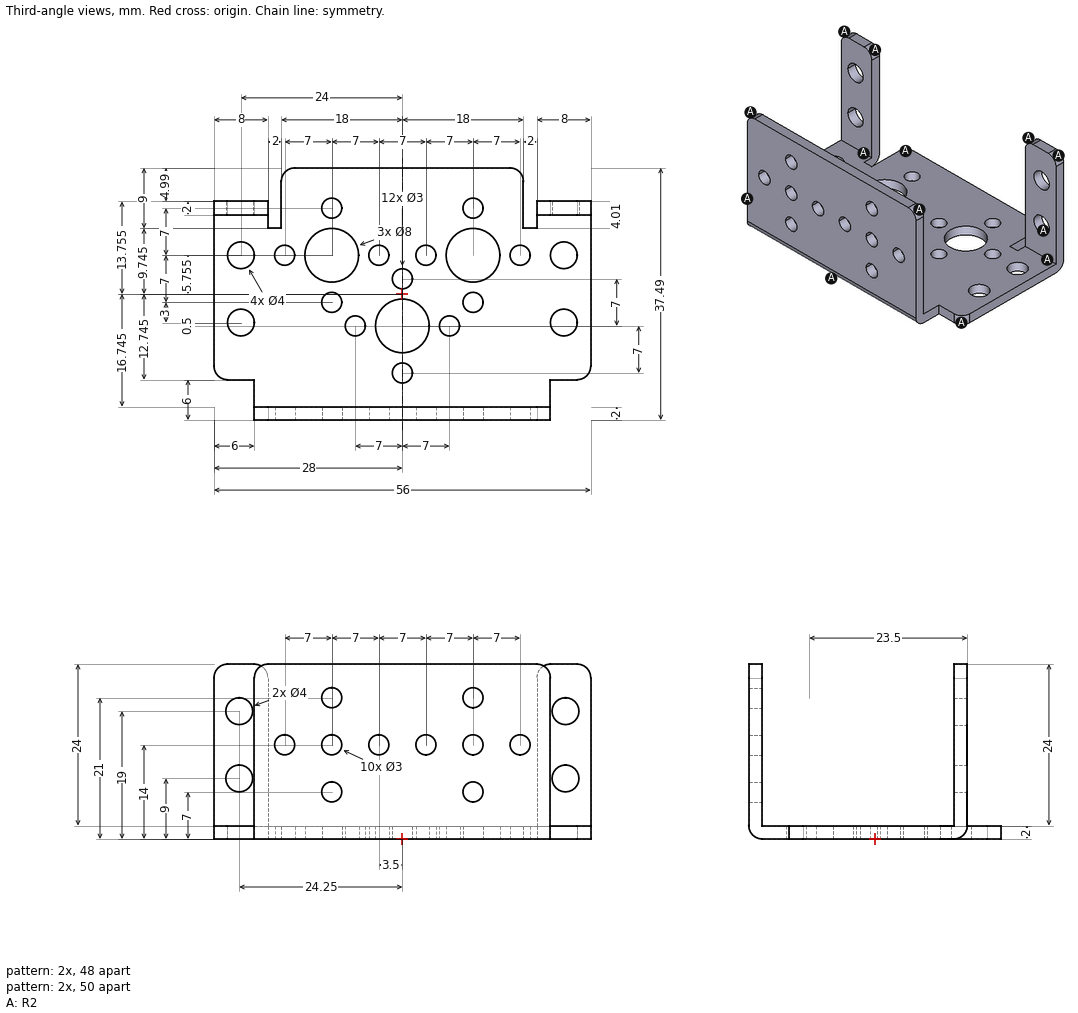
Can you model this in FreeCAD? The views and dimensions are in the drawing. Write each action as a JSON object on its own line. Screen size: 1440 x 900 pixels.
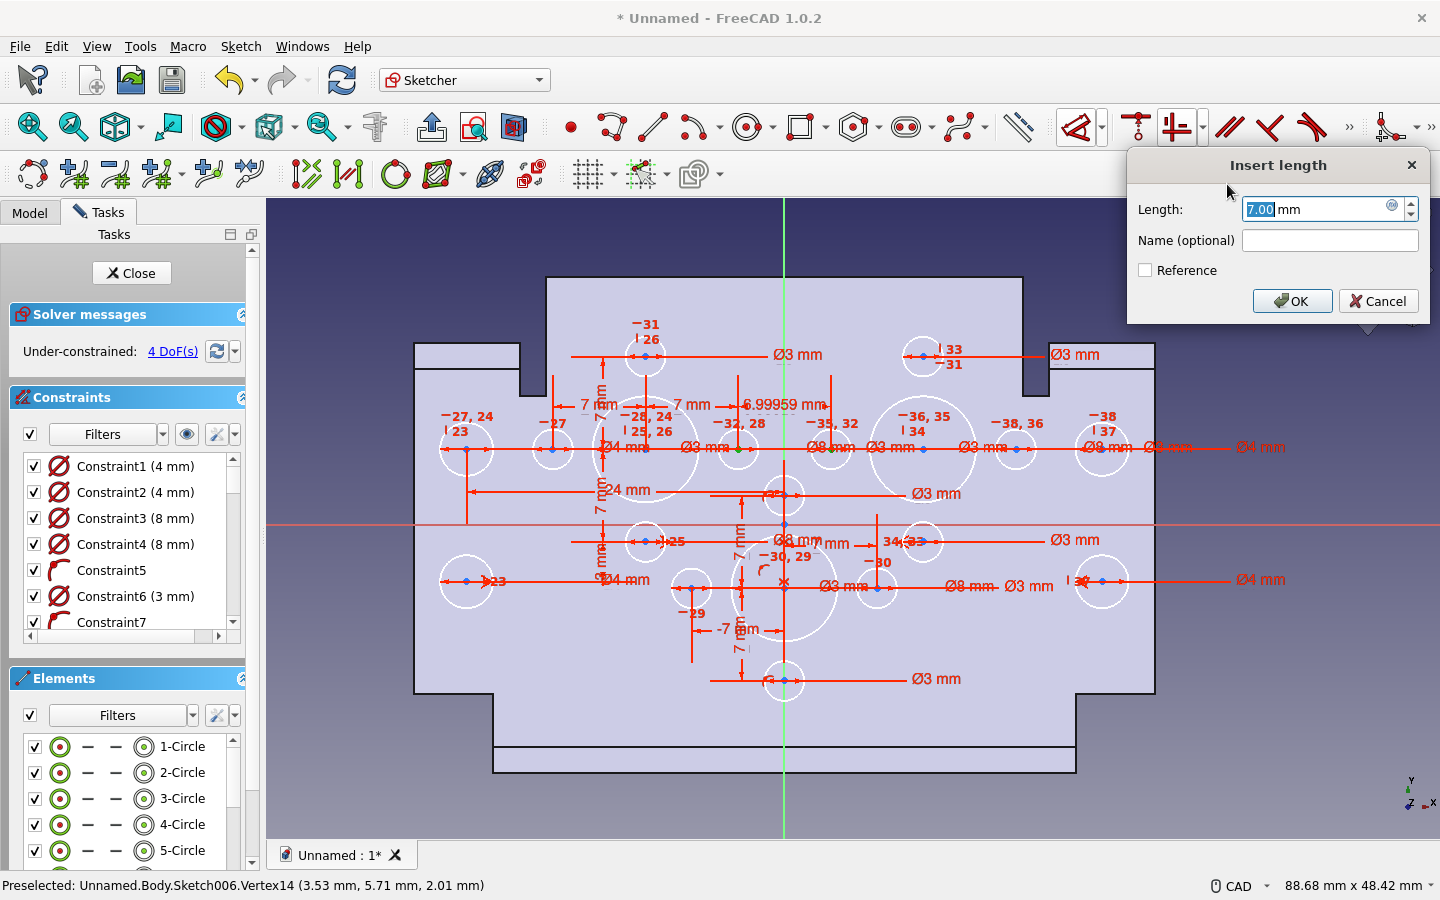
{"action": "type", "text": "7"}
{"action": "key", "text": "Return"}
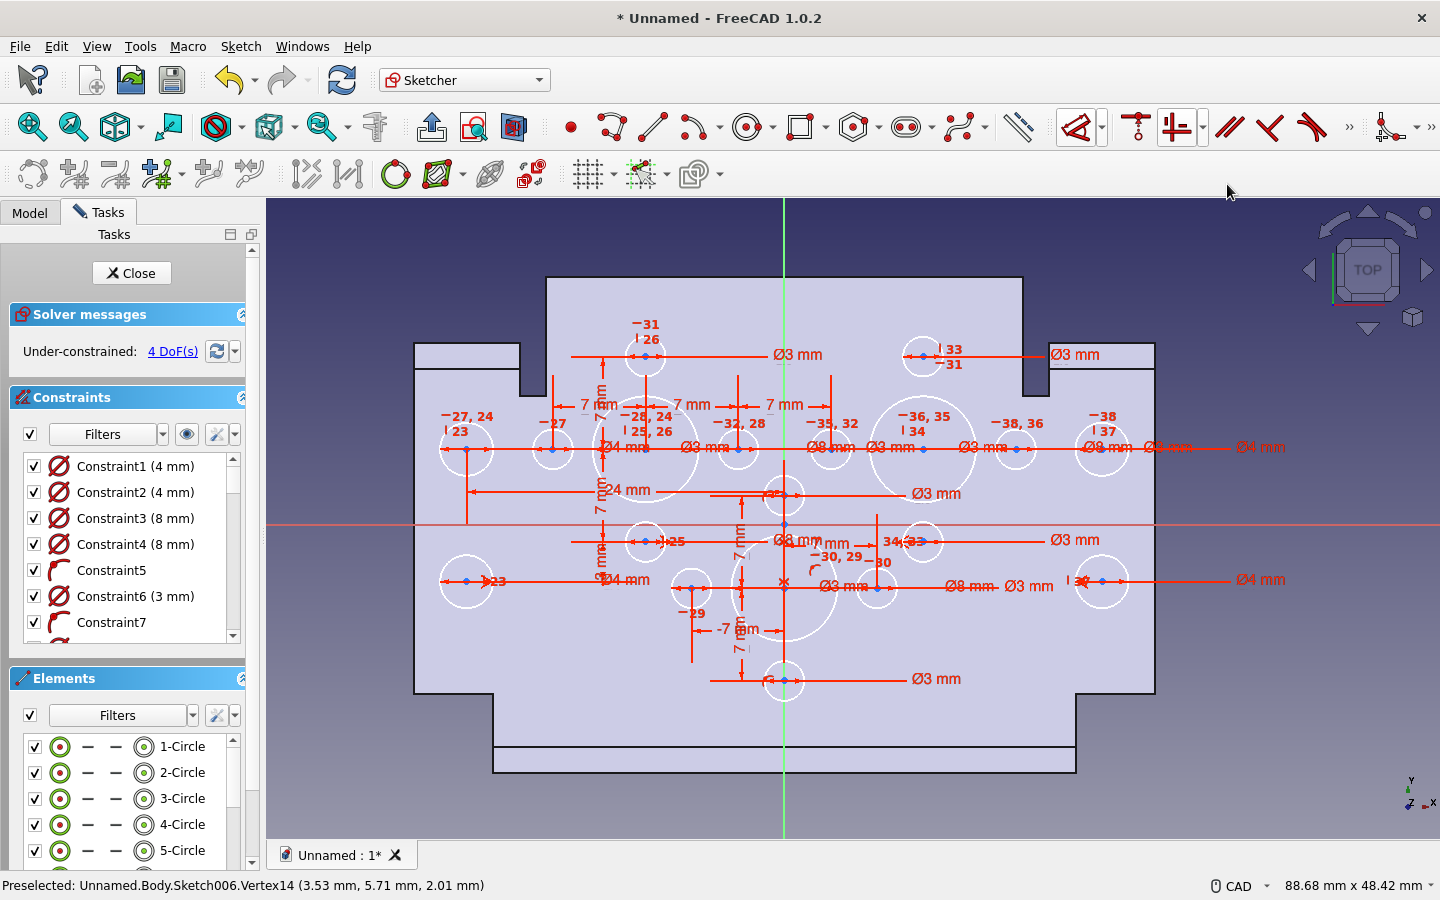
{"action": "left_click", "coordinate": [923, 357]}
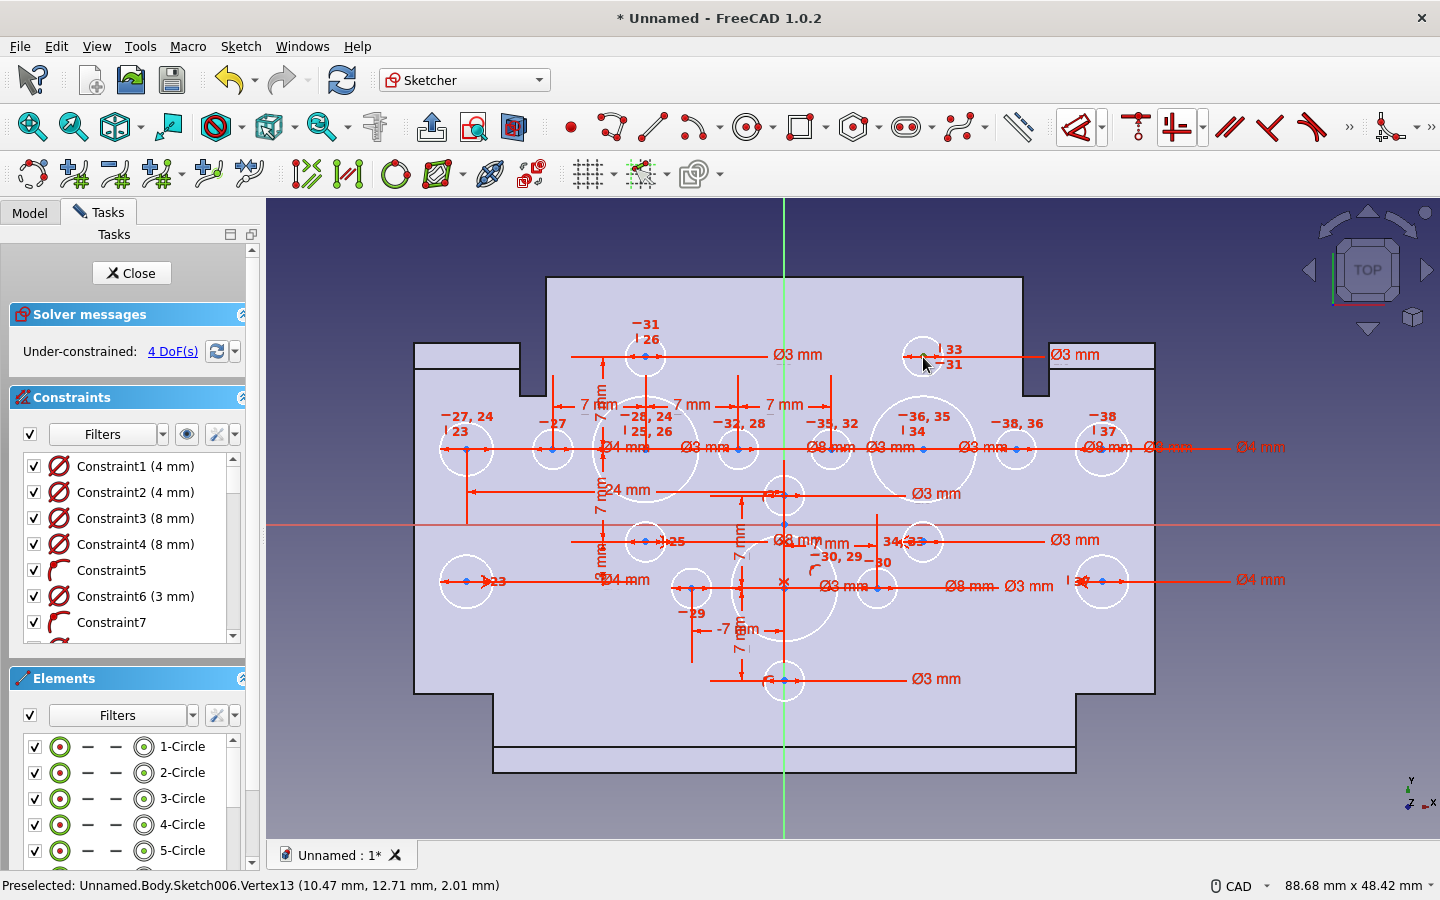
{"action": "left_click", "coordinate": [831, 449]}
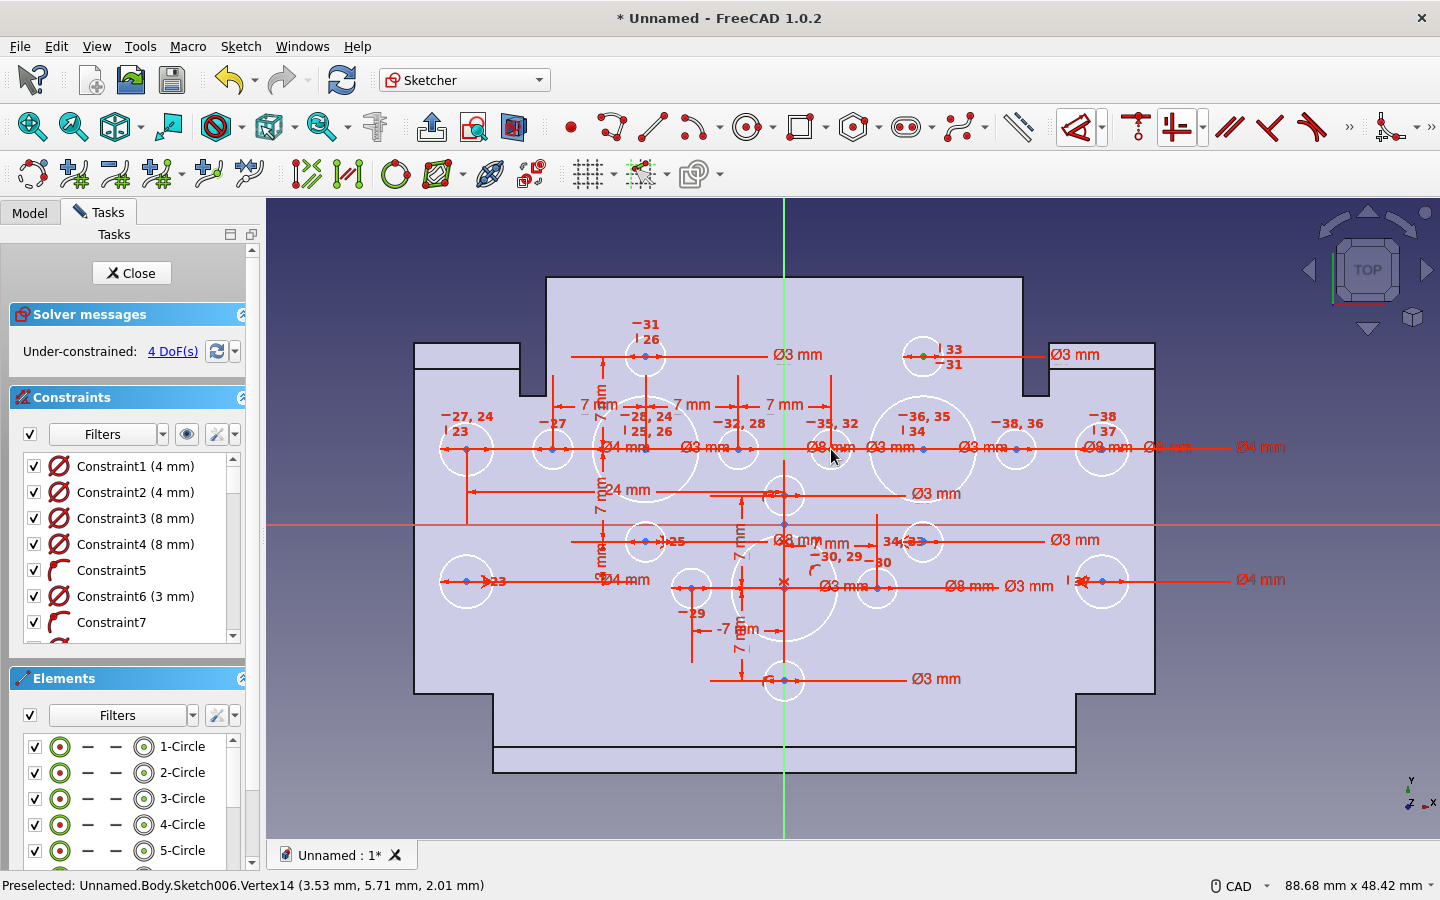
{"action": "left_click", "coordinate": [1102, 128]}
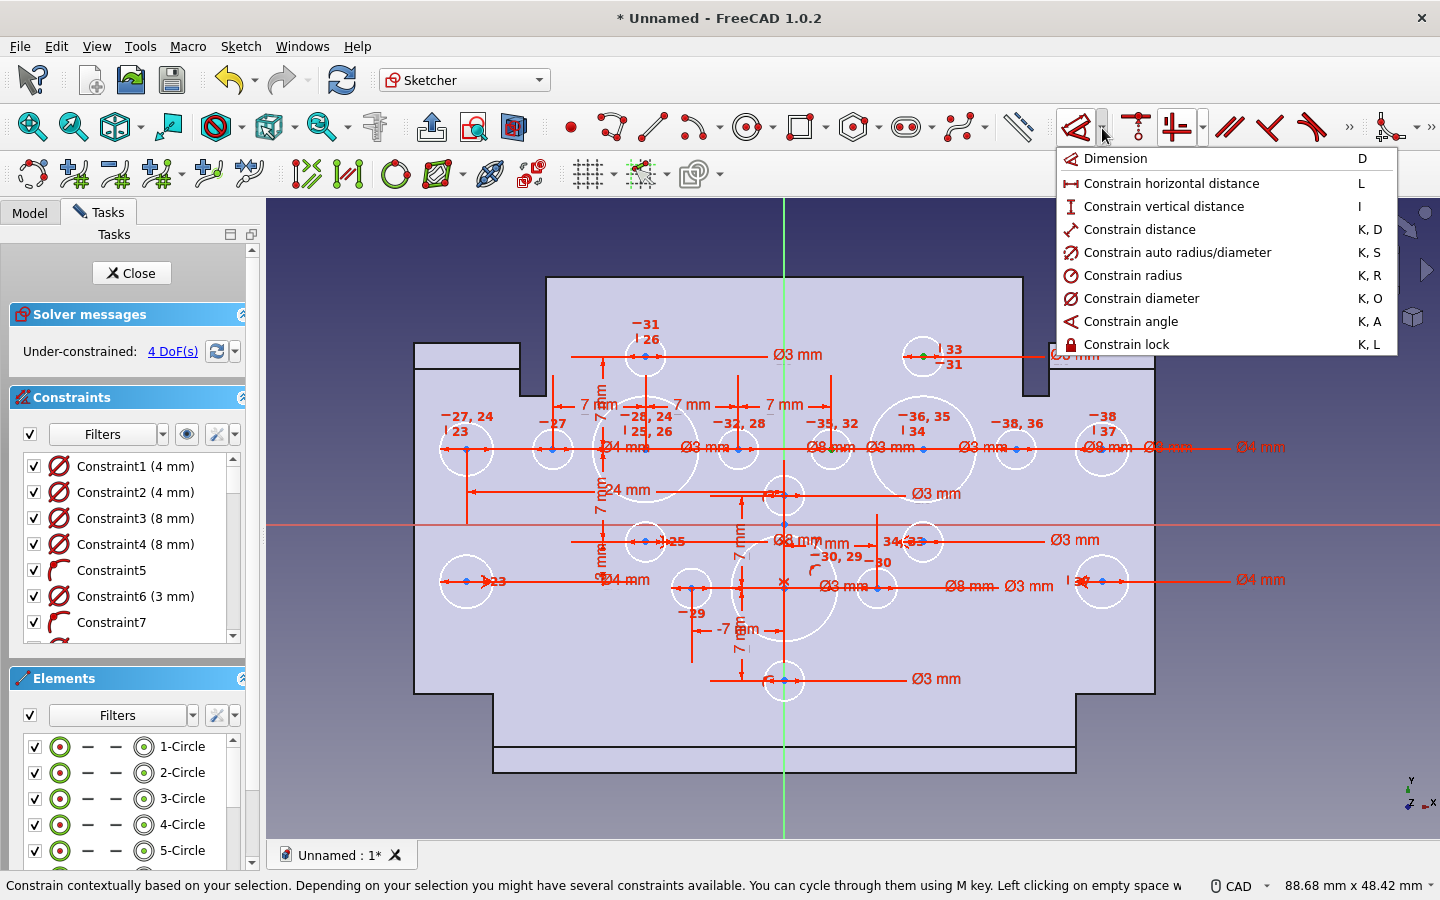
{"action": "left_click", "coordinate": [1227, 184]}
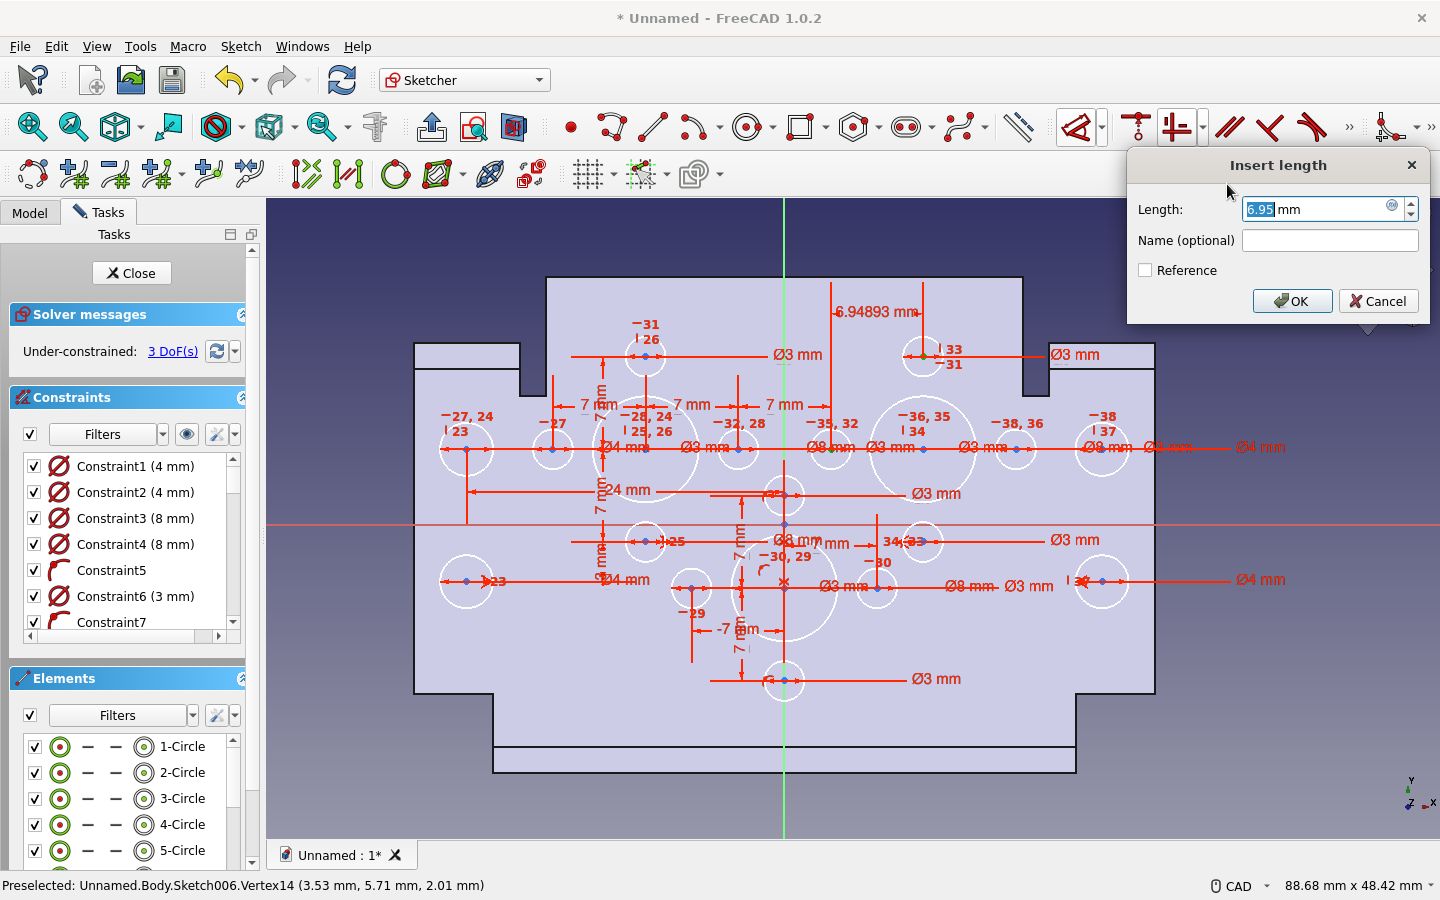
{"action": "type", "text": "7"}
{"action": "key", "text": "Return"}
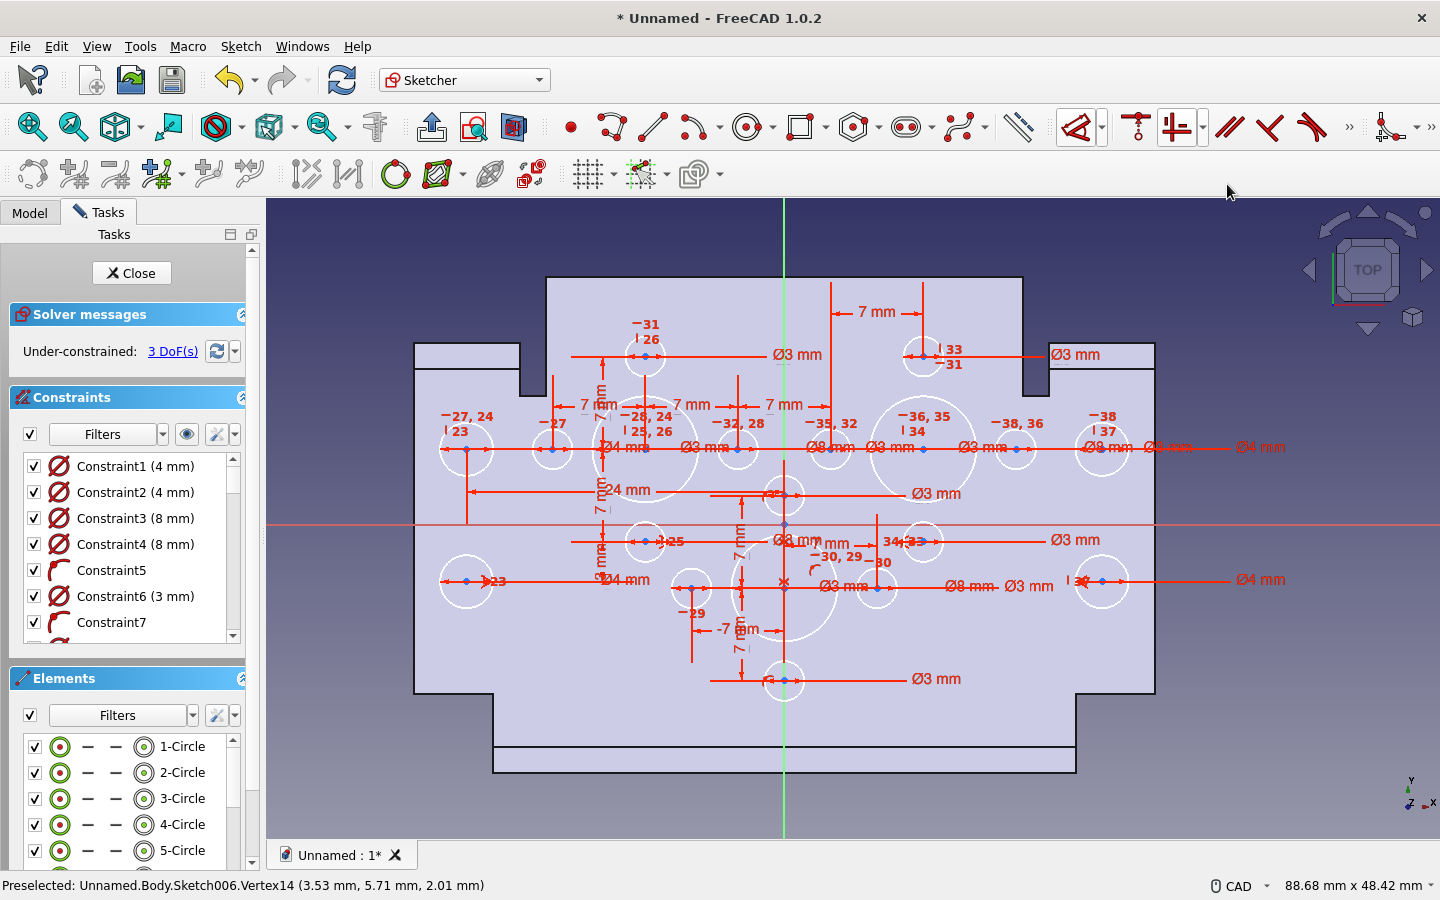
{"action": "left_click", "coordinate": [923, 449]}